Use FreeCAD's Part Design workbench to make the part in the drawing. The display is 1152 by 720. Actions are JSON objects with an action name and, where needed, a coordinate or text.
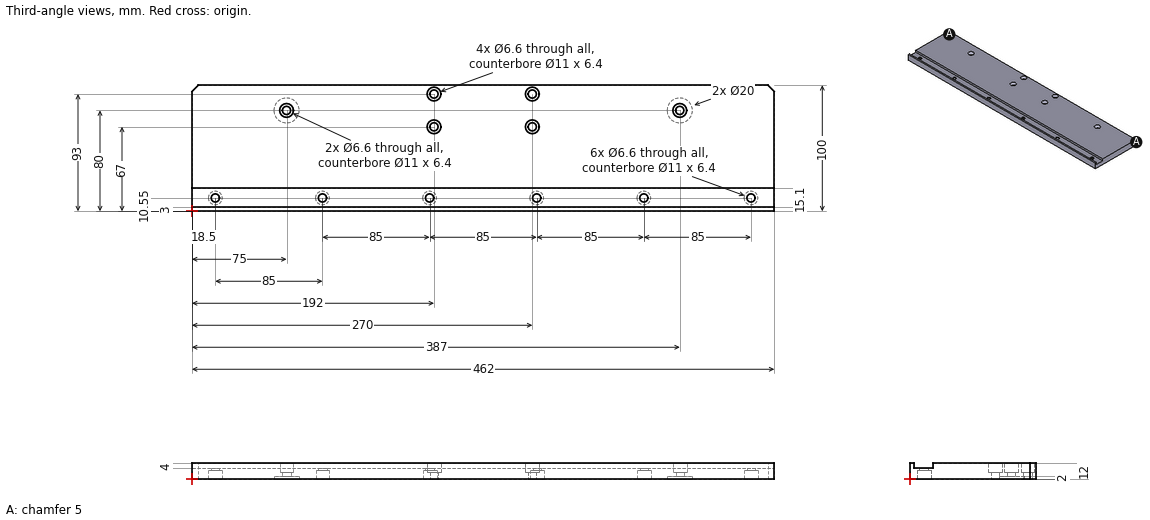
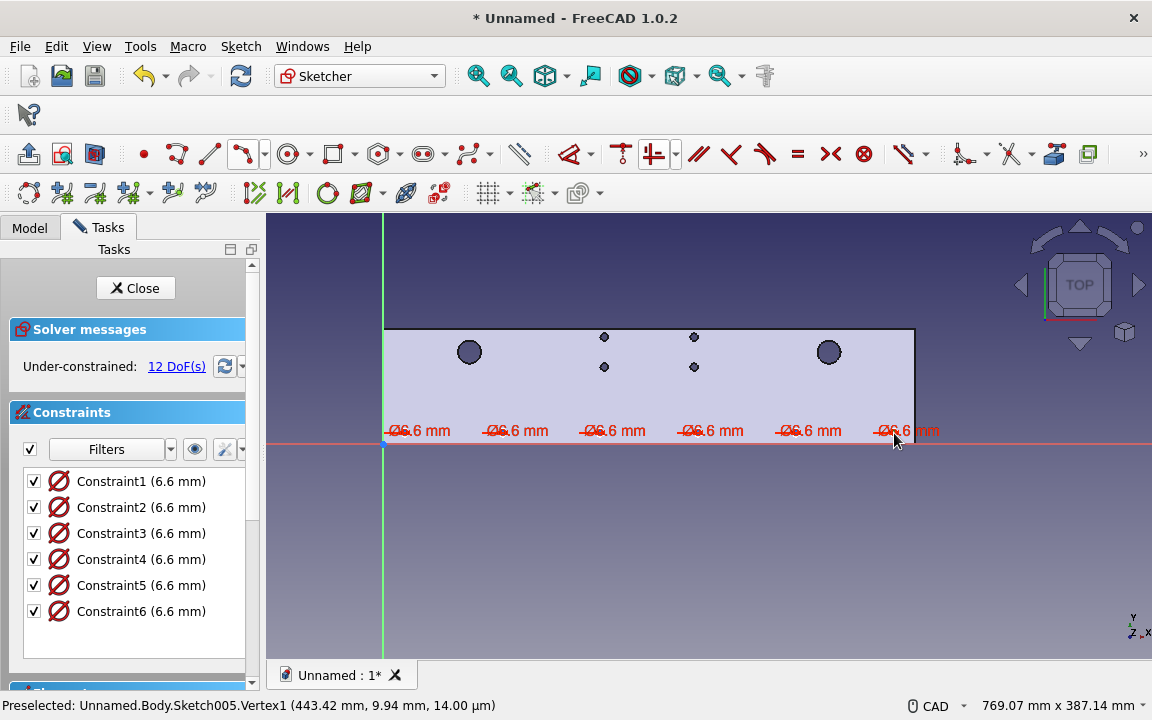
{"action": "left_click", "coordinate": [796, 433]}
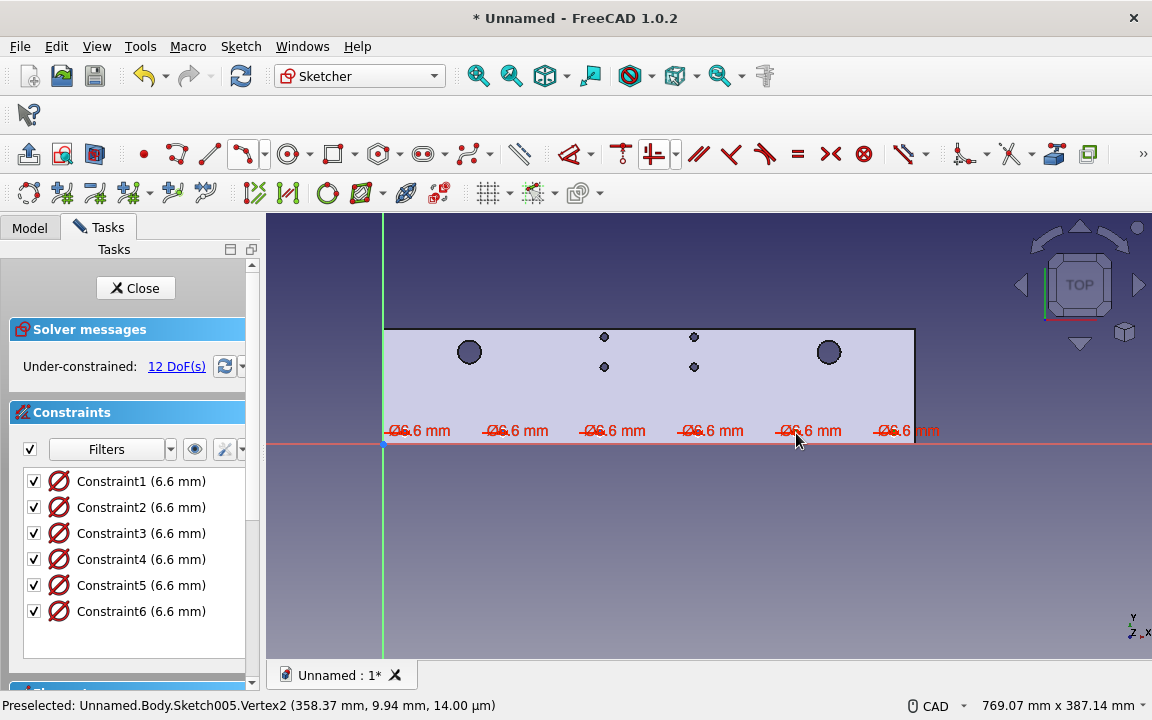
{"action": "left_click", "coordinate": [676, 154]}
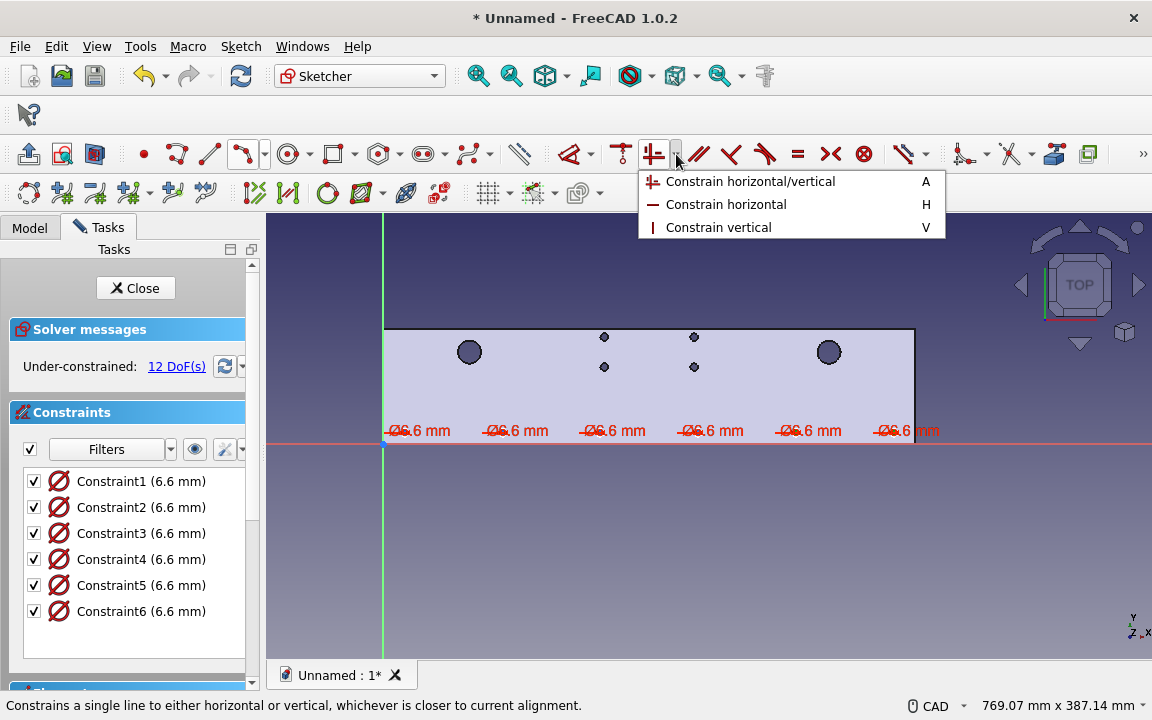
{"action": "left_click", "coordinate": [792, 204]}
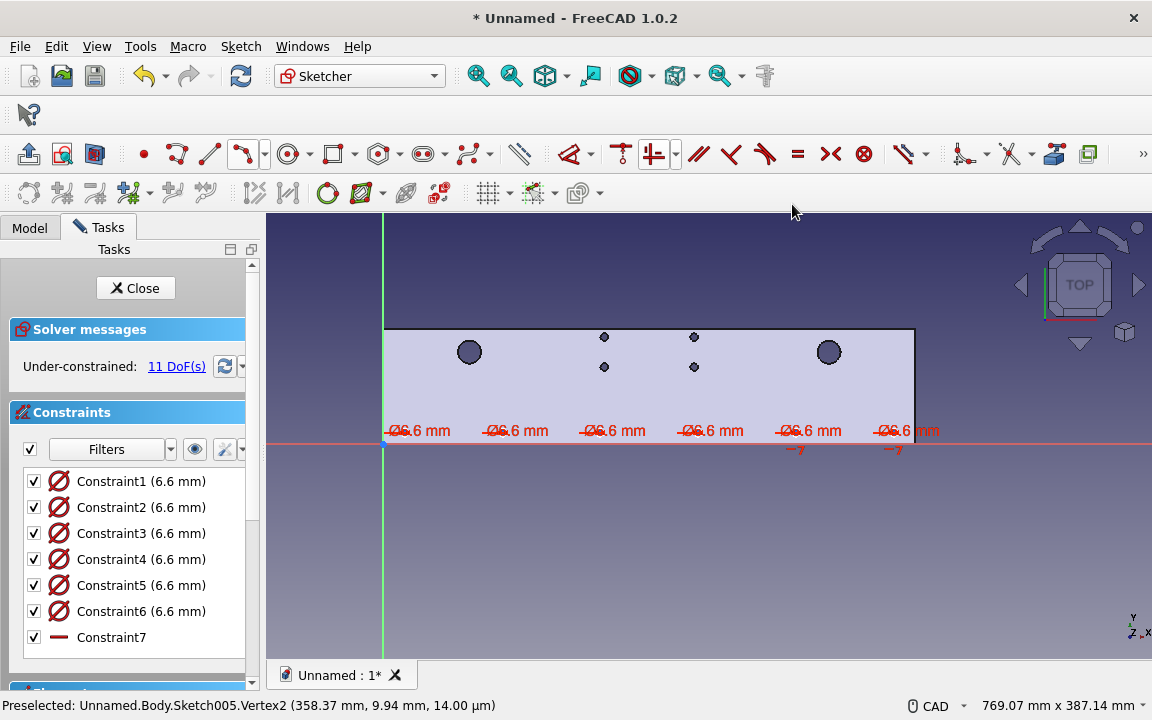
{"action": "left_click", "coordinate": [796, 433]}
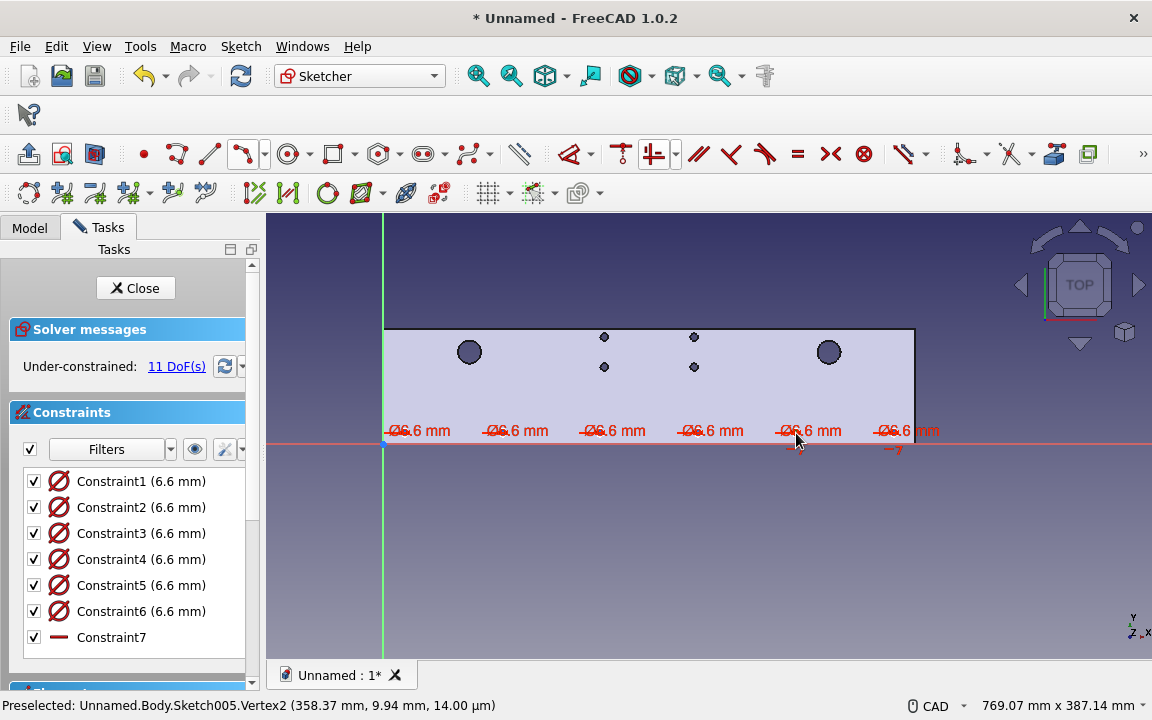
{"action": "left_click", "coordinate": [698, 433]}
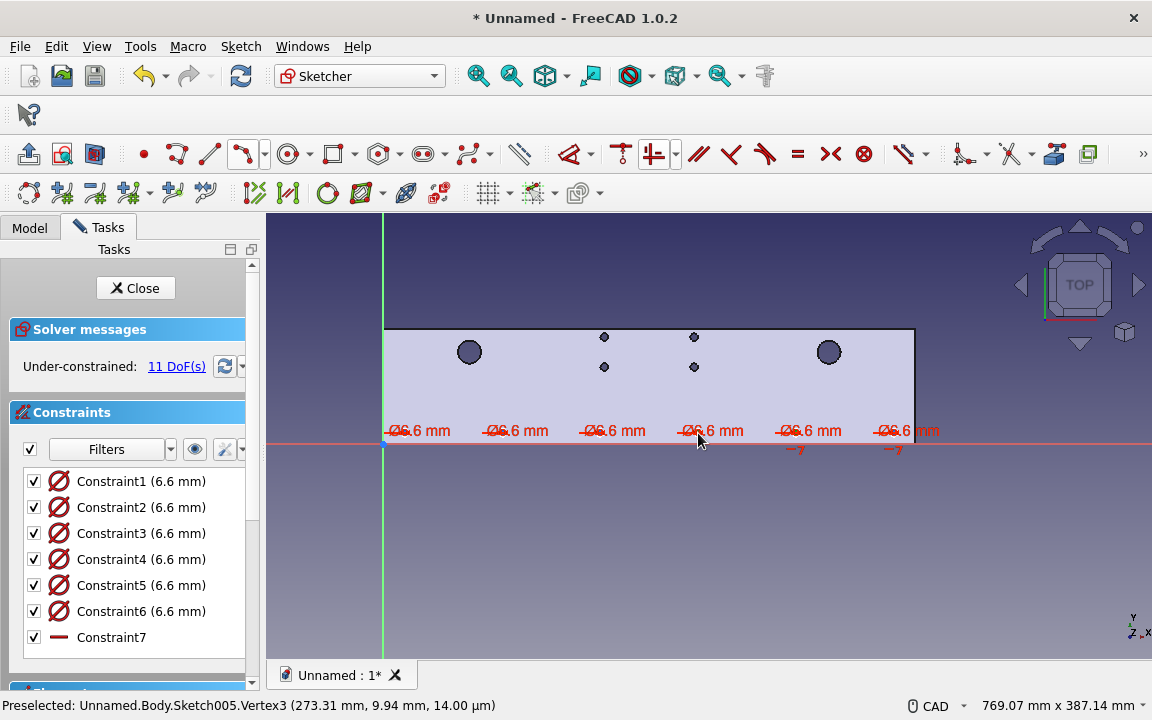
{"action": "key", "text": "h"}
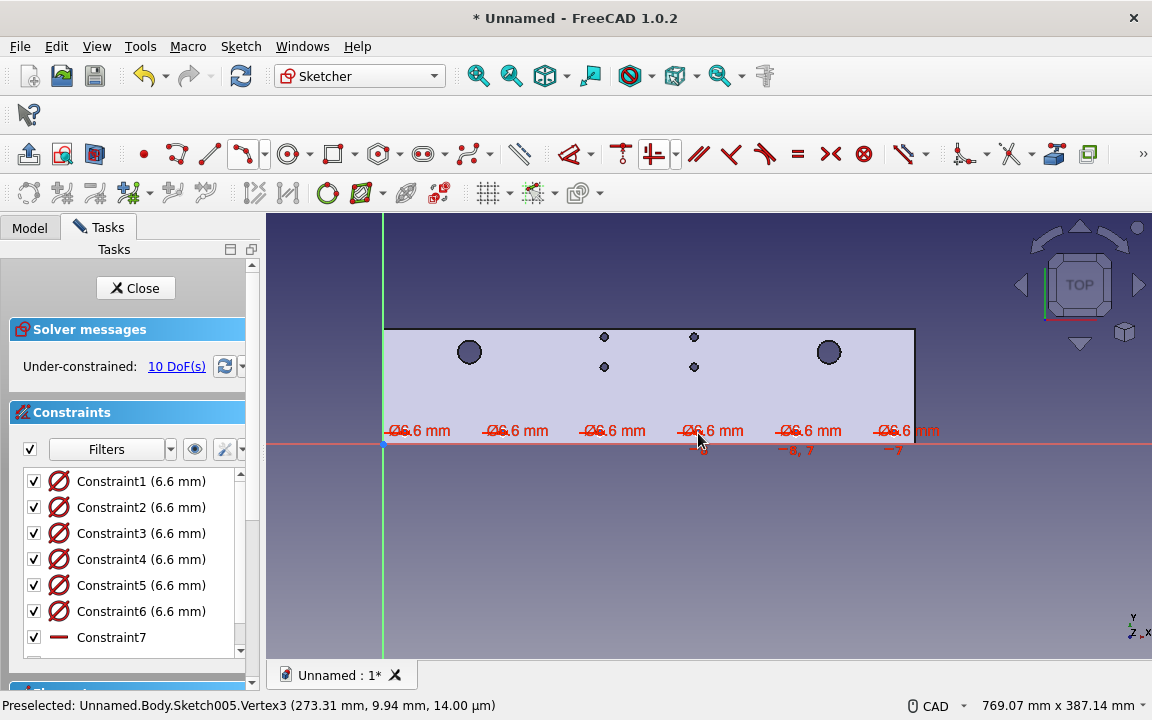
{"action": "left_click", "coordinate": [698, 433]}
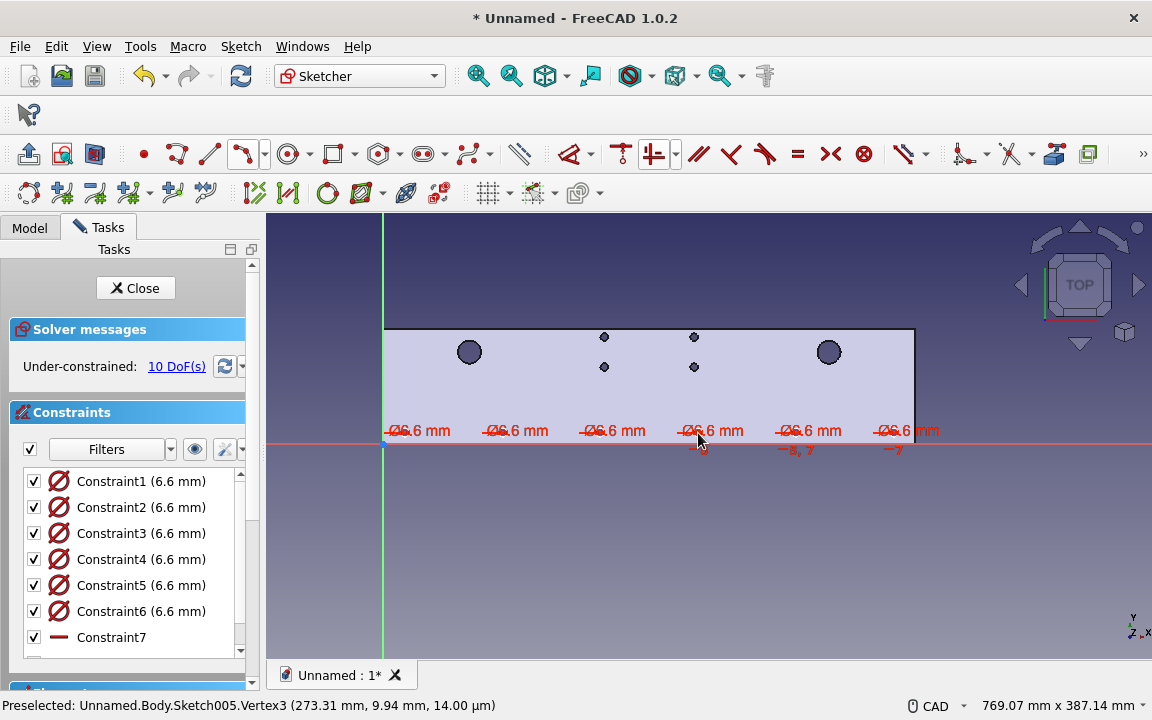
{"action": "left_click", "coordinate": [600, 433]}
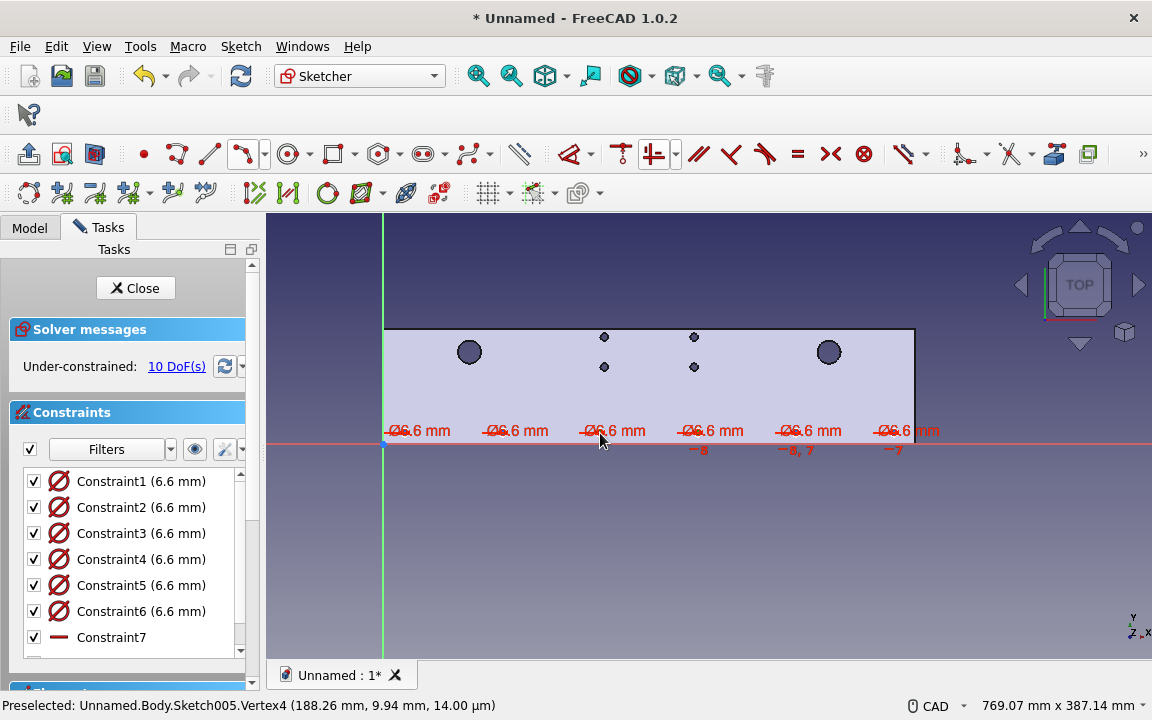
{"action": "key", "text": "h"}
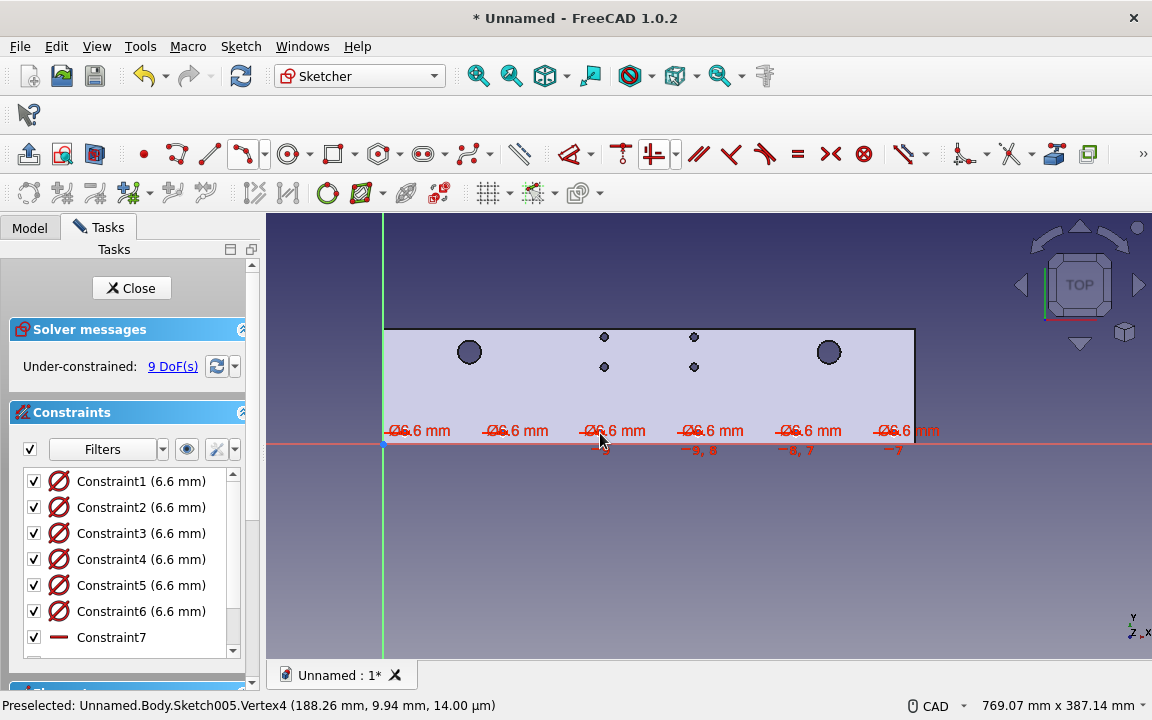
{"action": "left_click", "coordinate": [600, 433]}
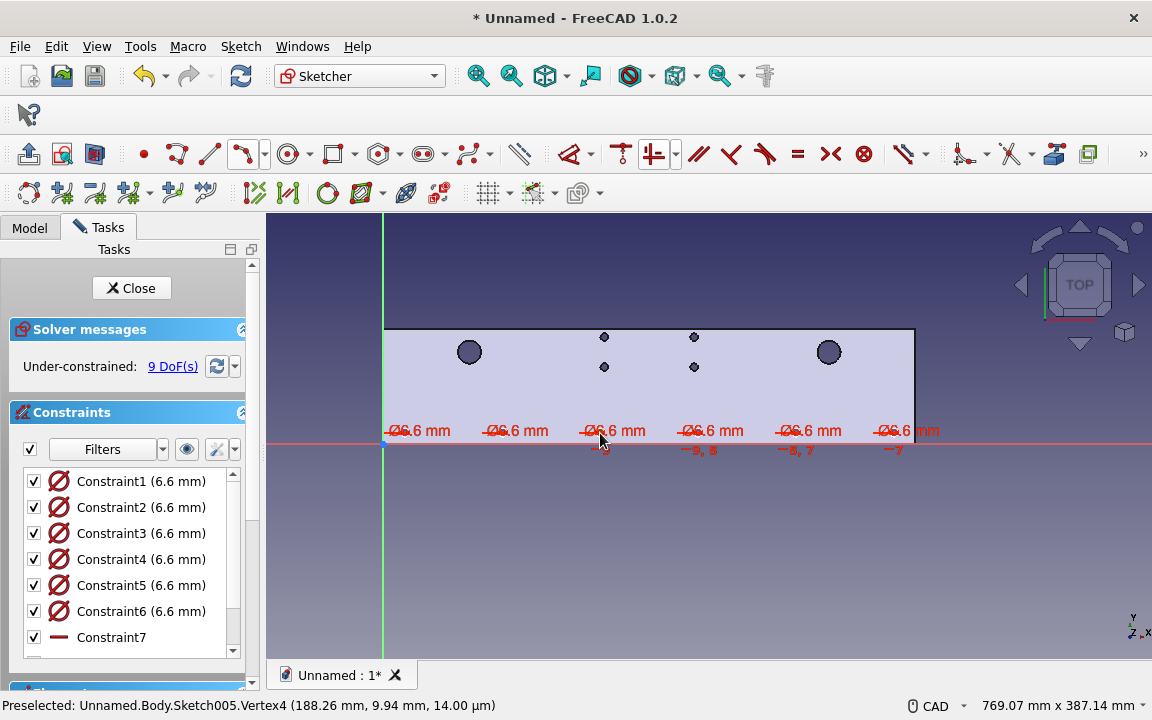
{"action": "left_click", "coordinate": [503, 433]}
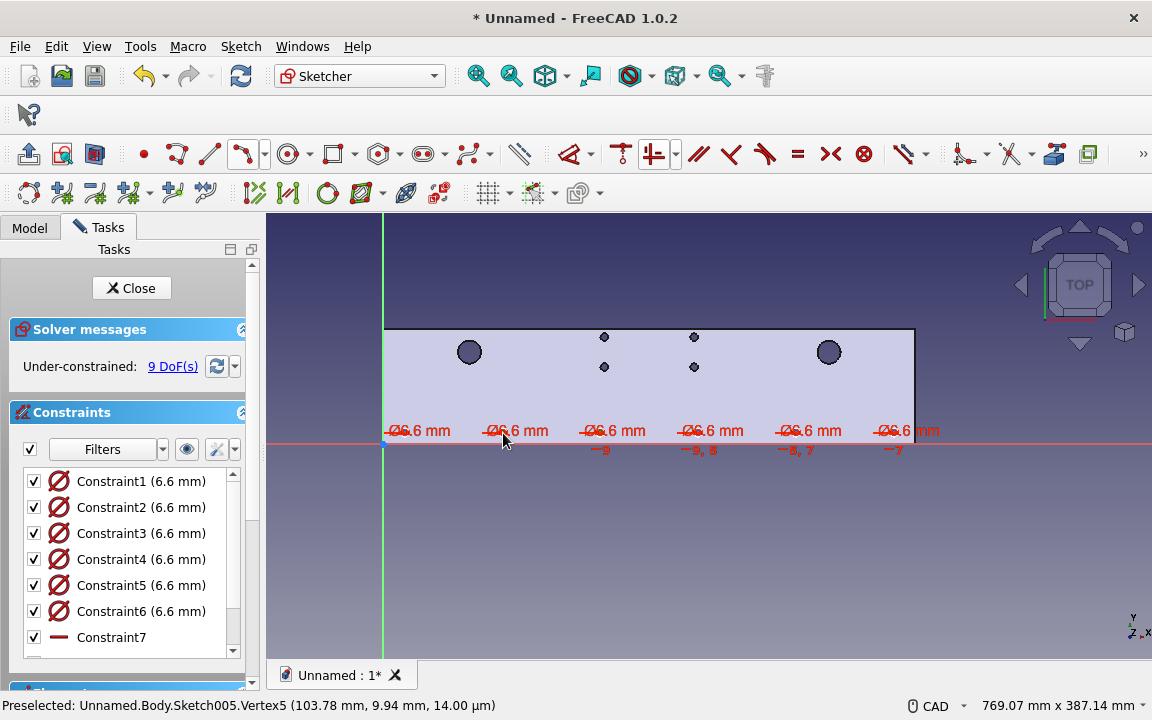
{"action": "key", "text": "h"}